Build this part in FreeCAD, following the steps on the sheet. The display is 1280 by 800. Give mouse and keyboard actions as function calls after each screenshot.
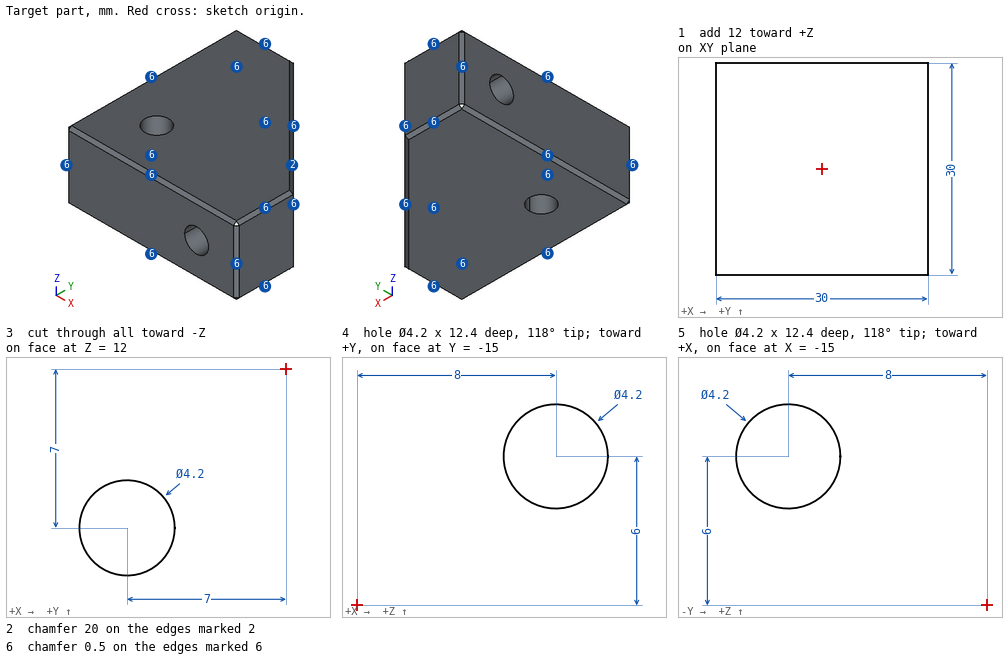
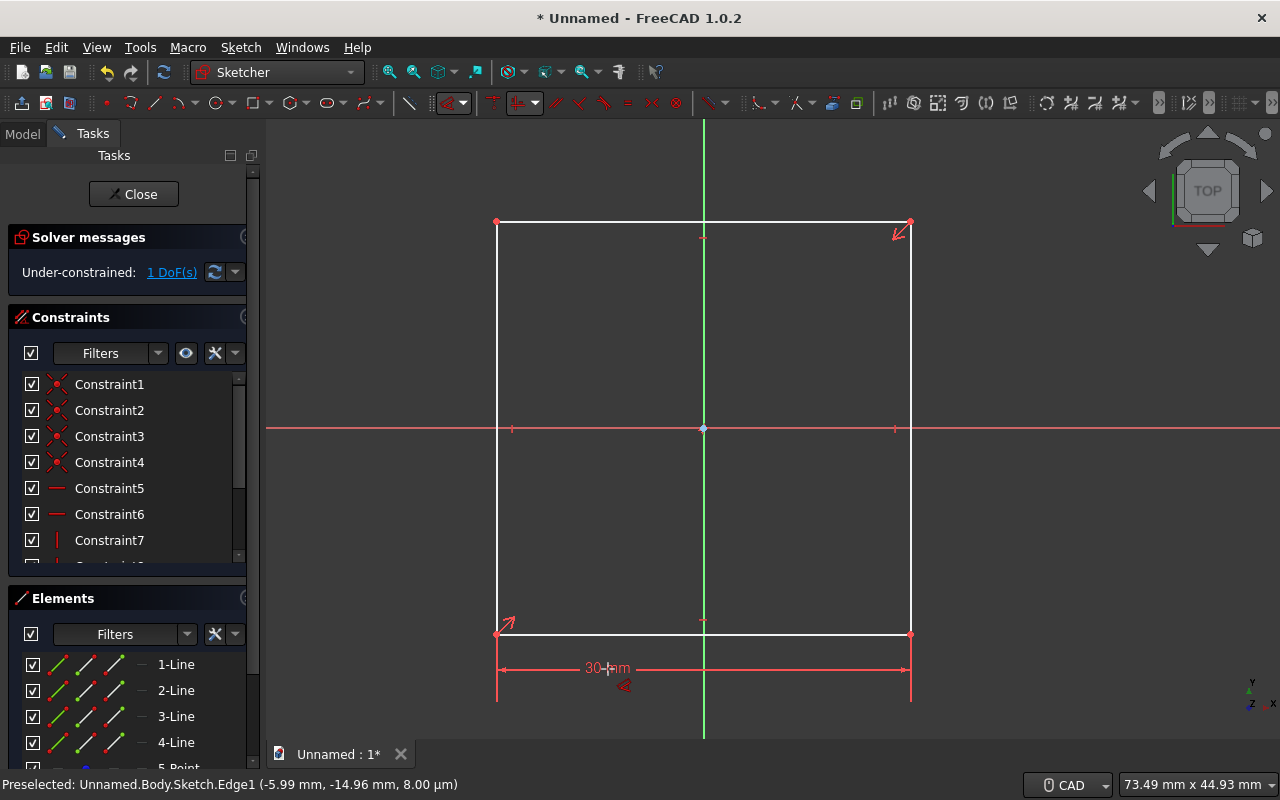
click(911, 511)
click(945, 333)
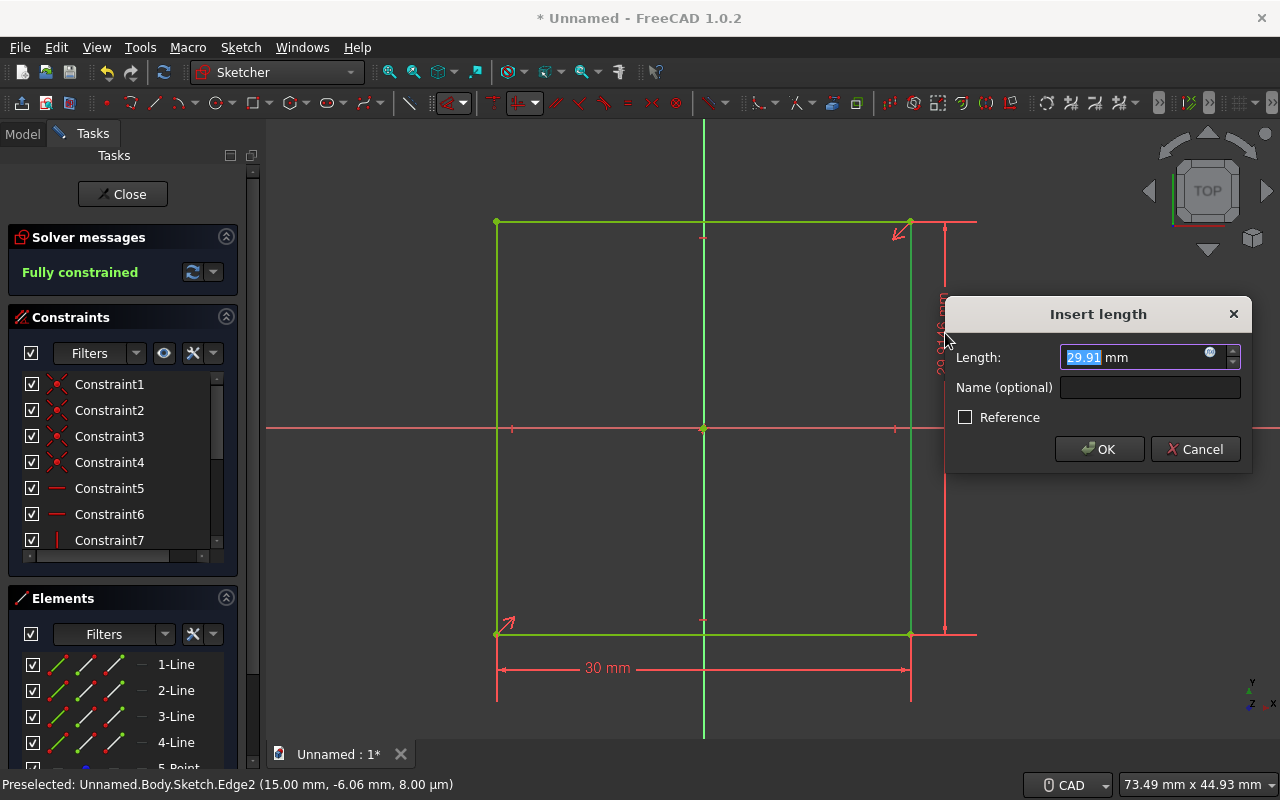
text(30)
key(Return)
key(Escape)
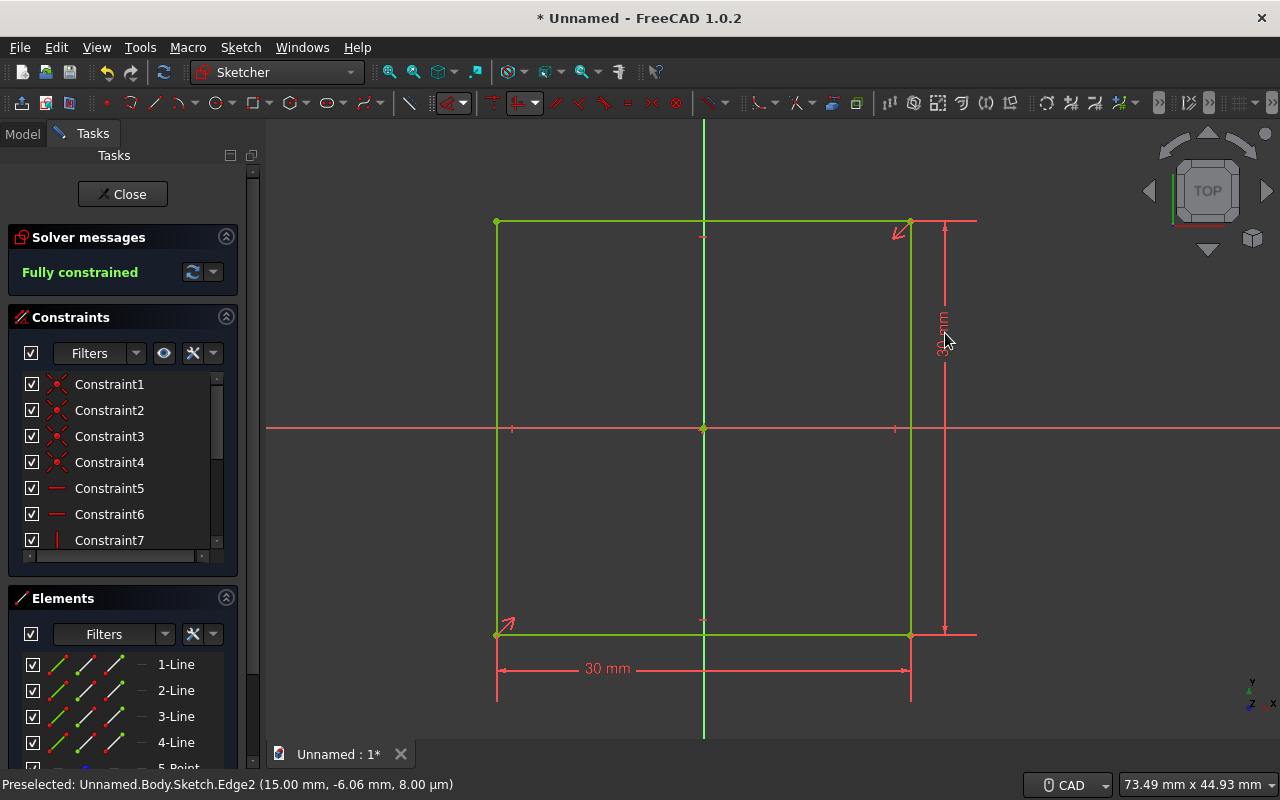
click(123, 194)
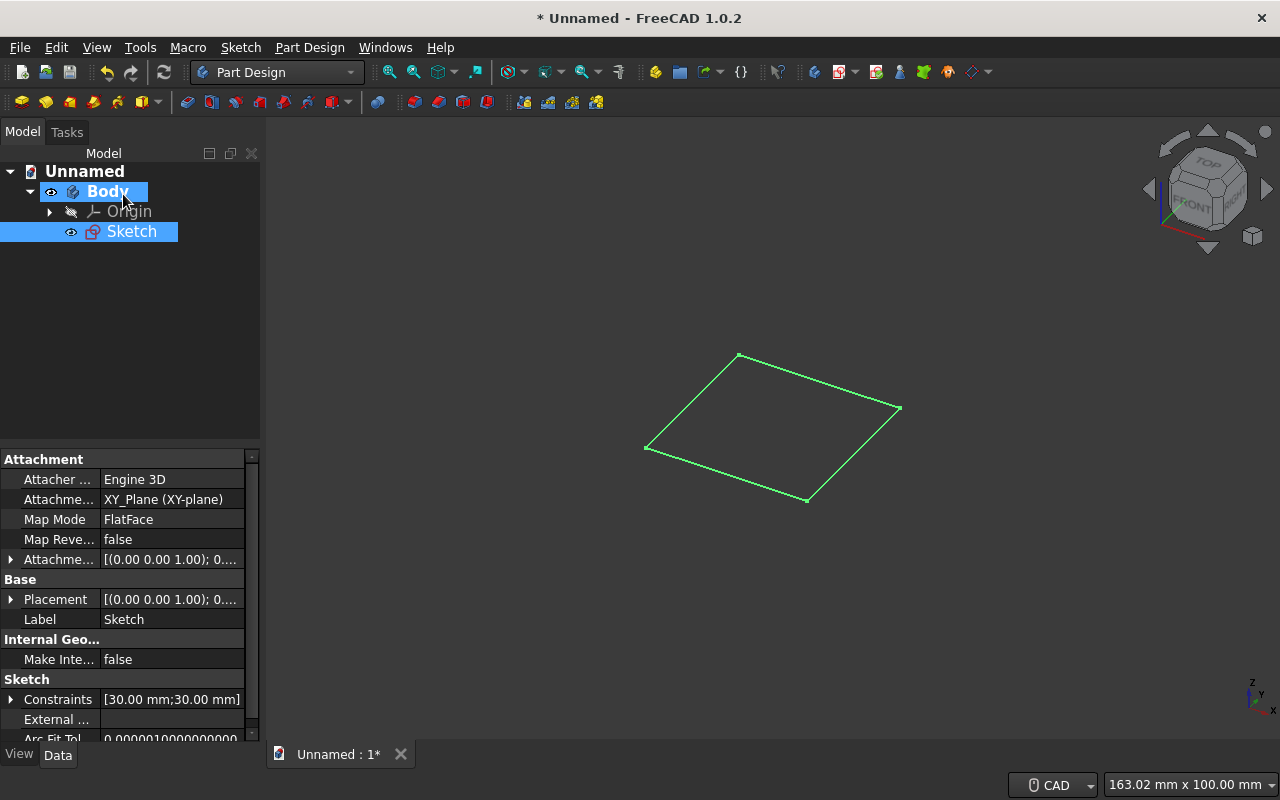
click(22, 102)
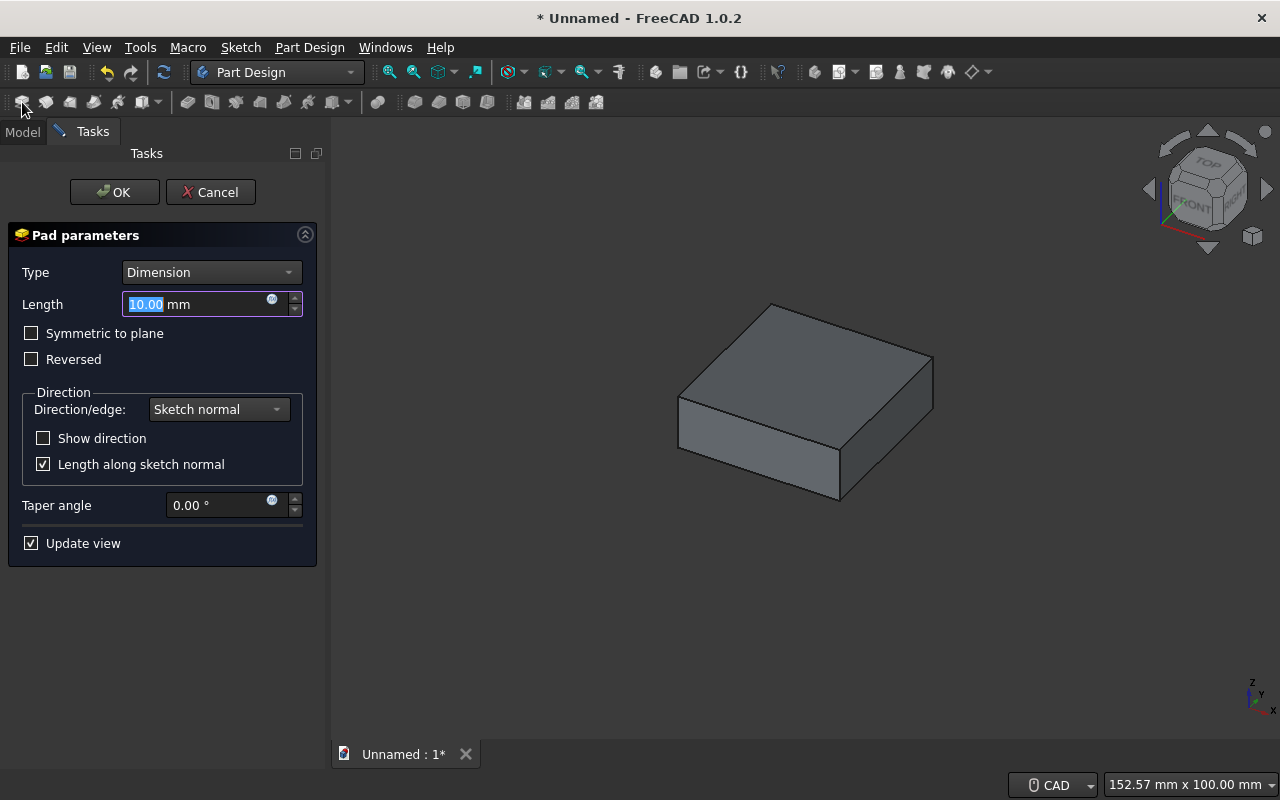
text(12)
key(Tab)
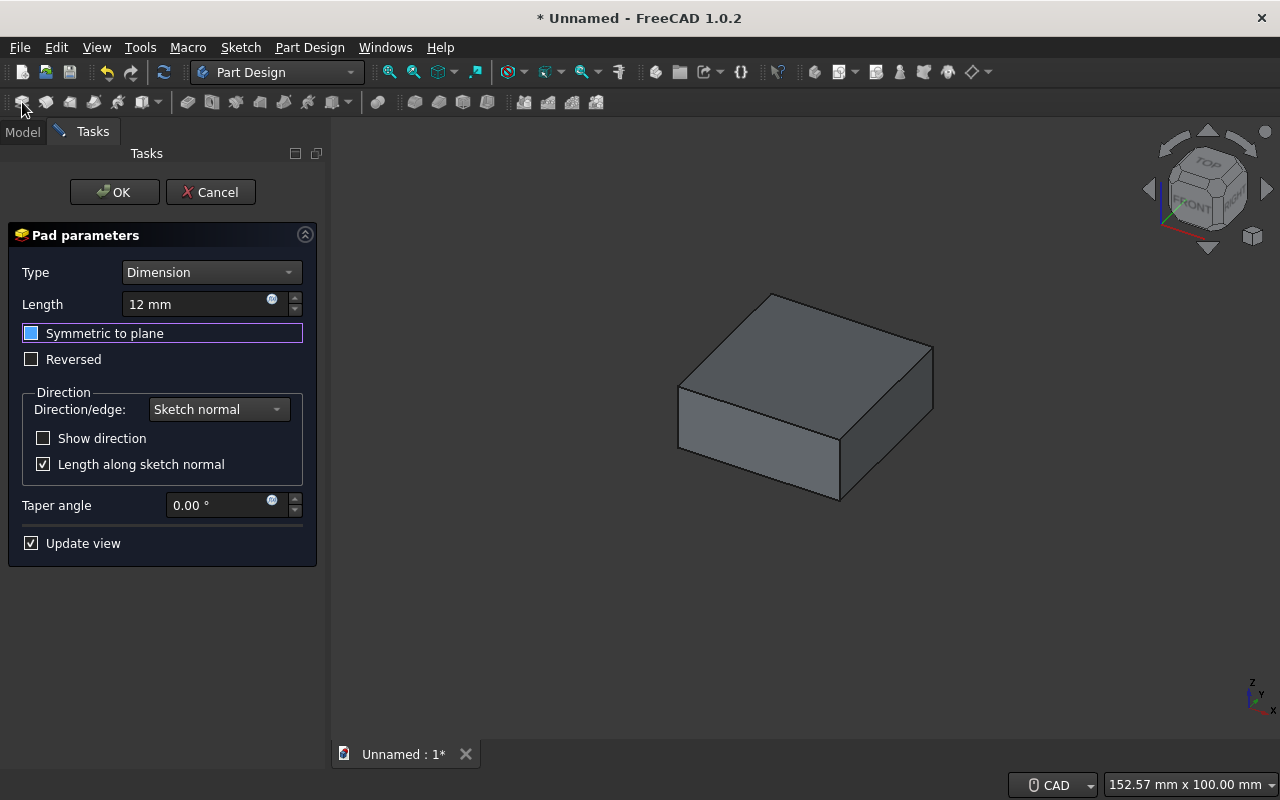
click(115, 192)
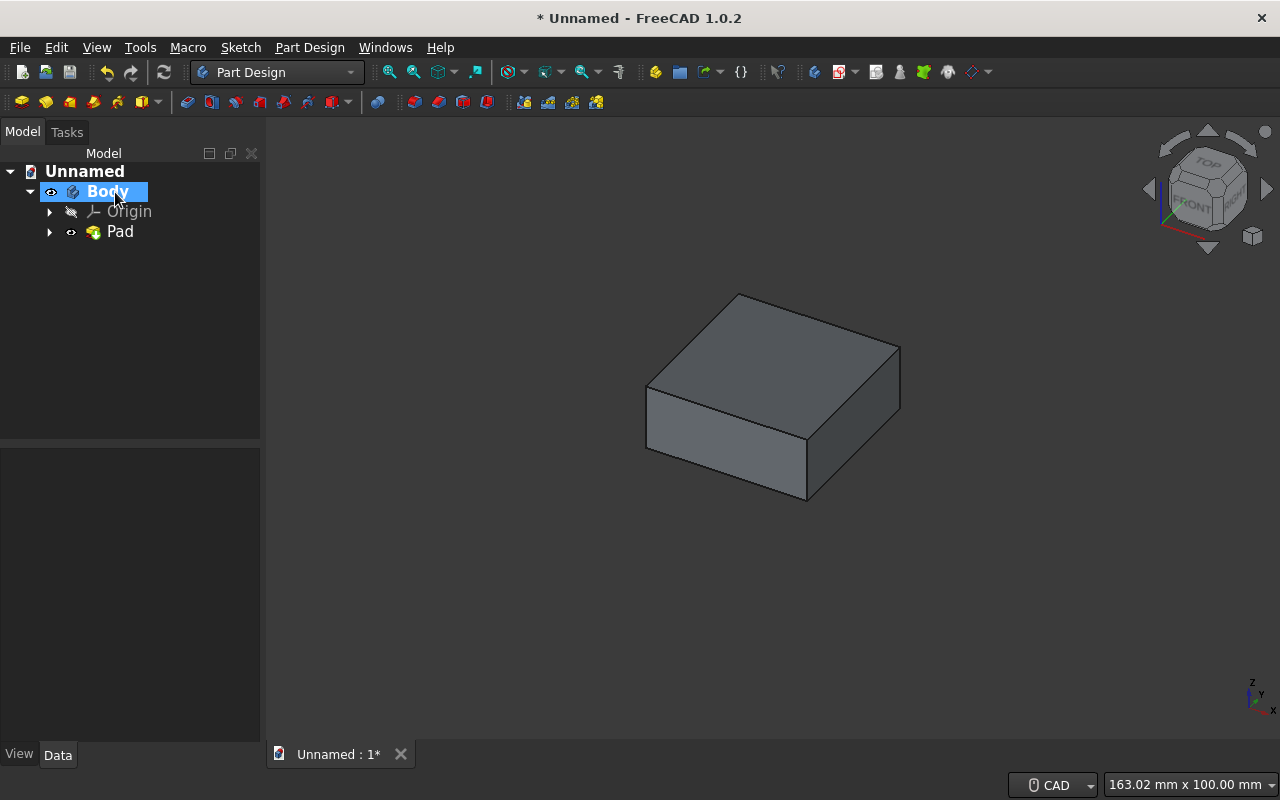
key(v)
key(f)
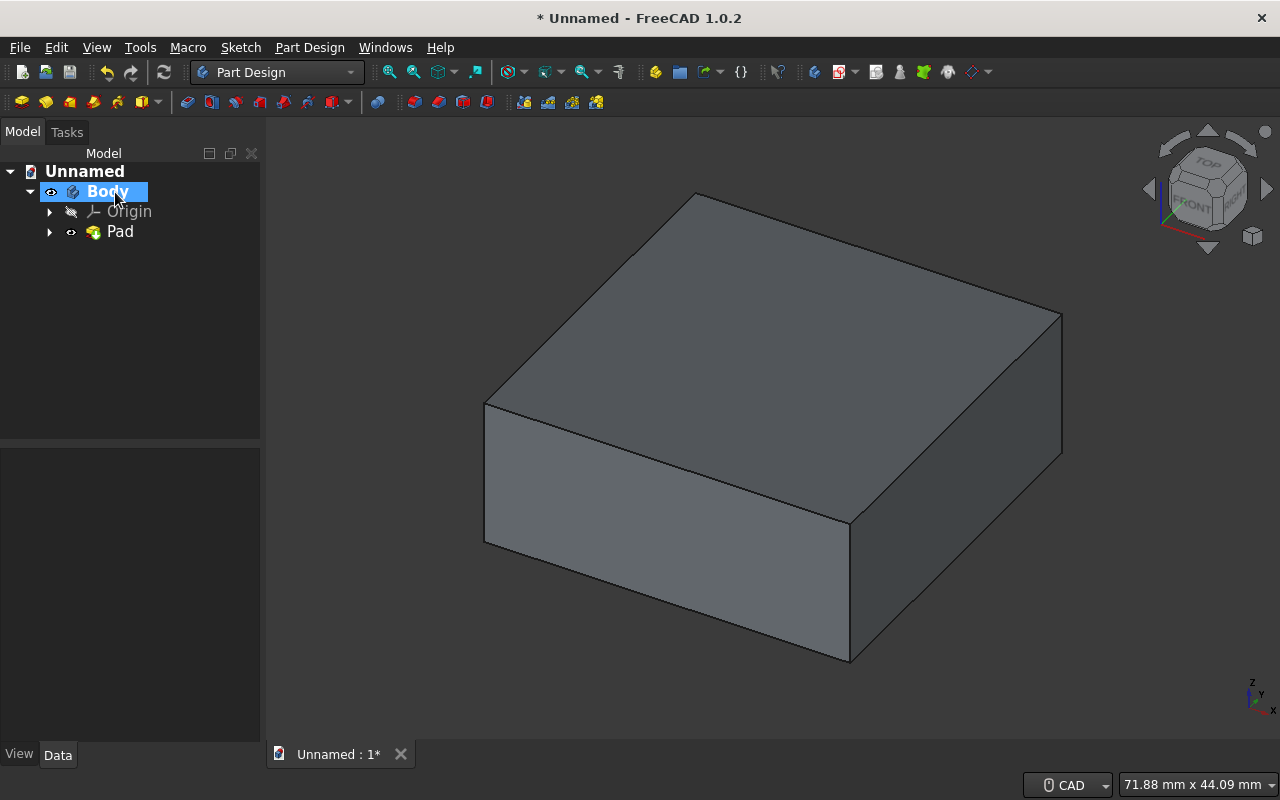
key(0)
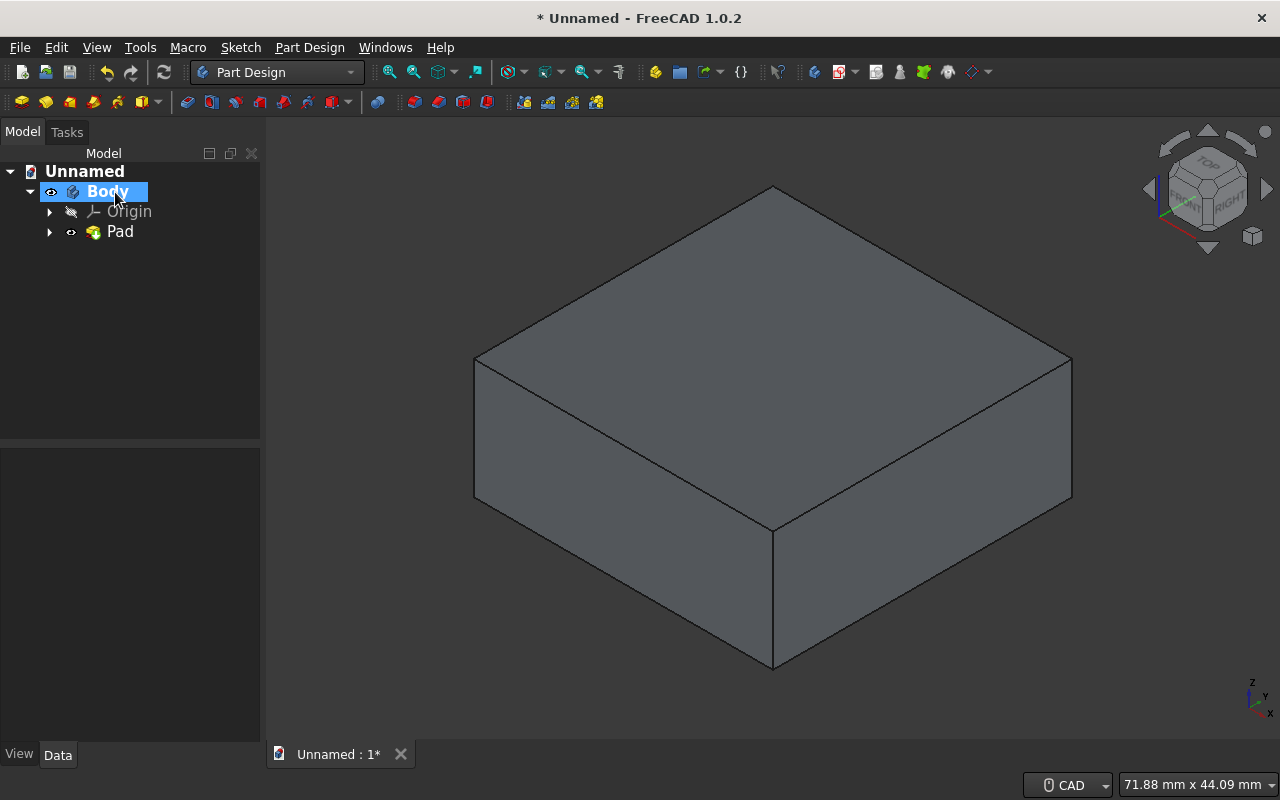
key(2)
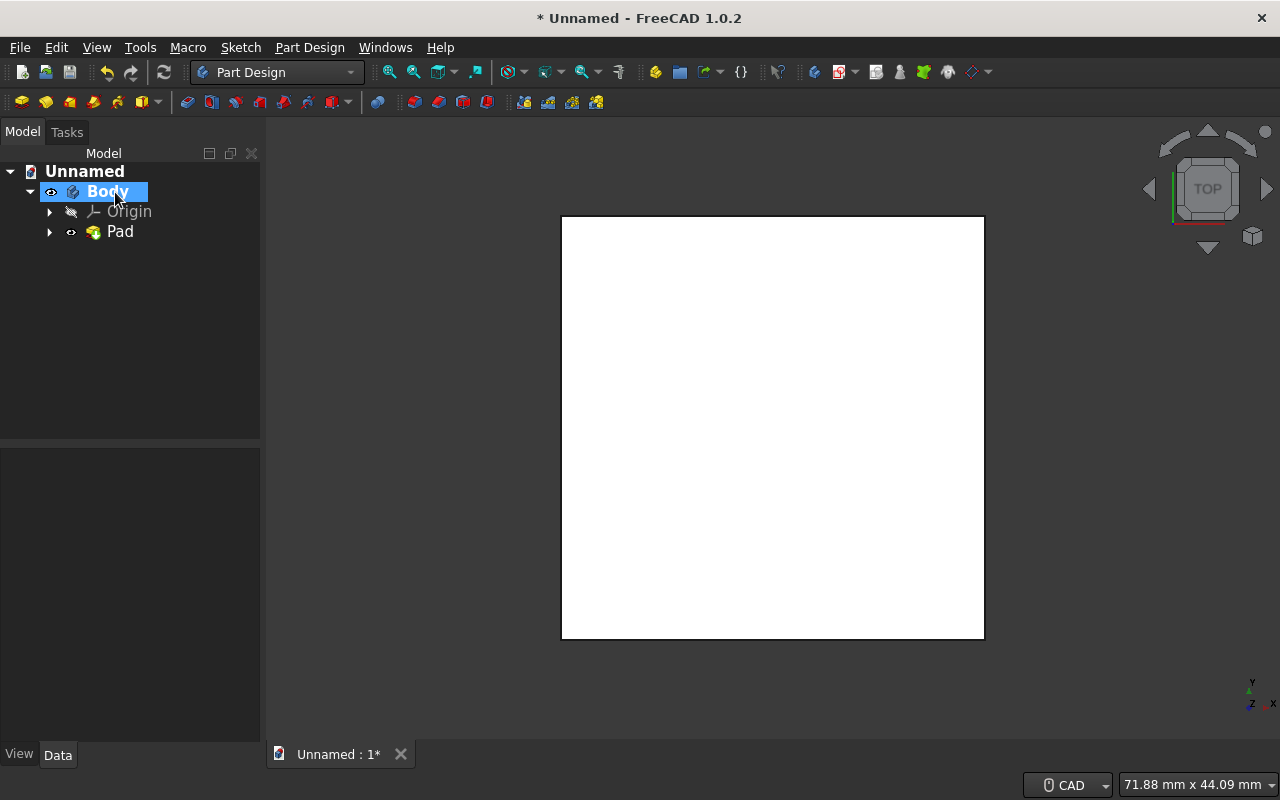
key(1)